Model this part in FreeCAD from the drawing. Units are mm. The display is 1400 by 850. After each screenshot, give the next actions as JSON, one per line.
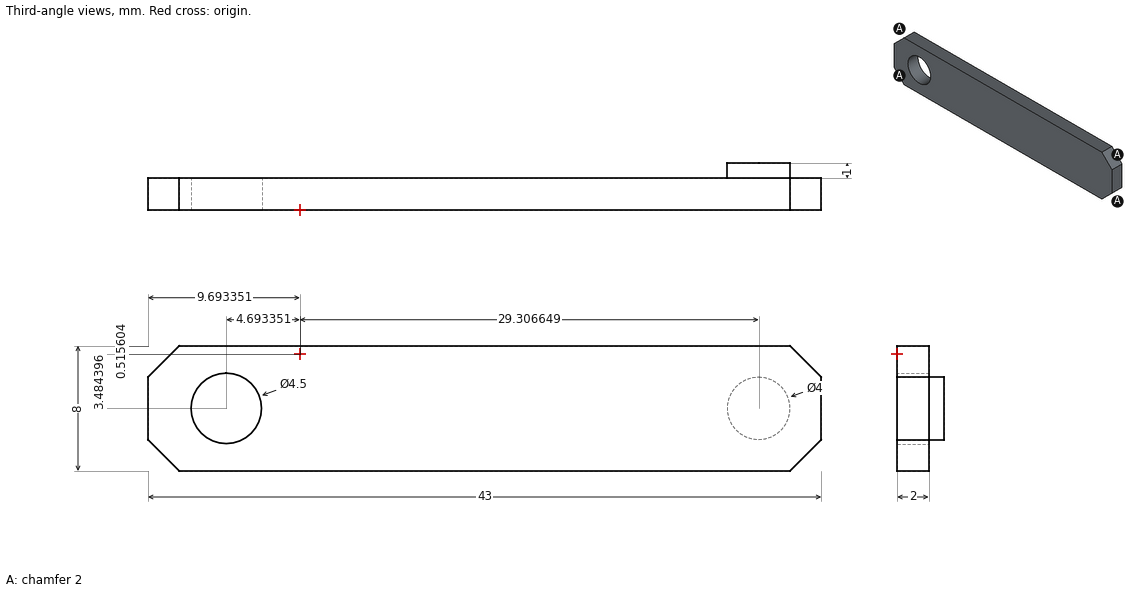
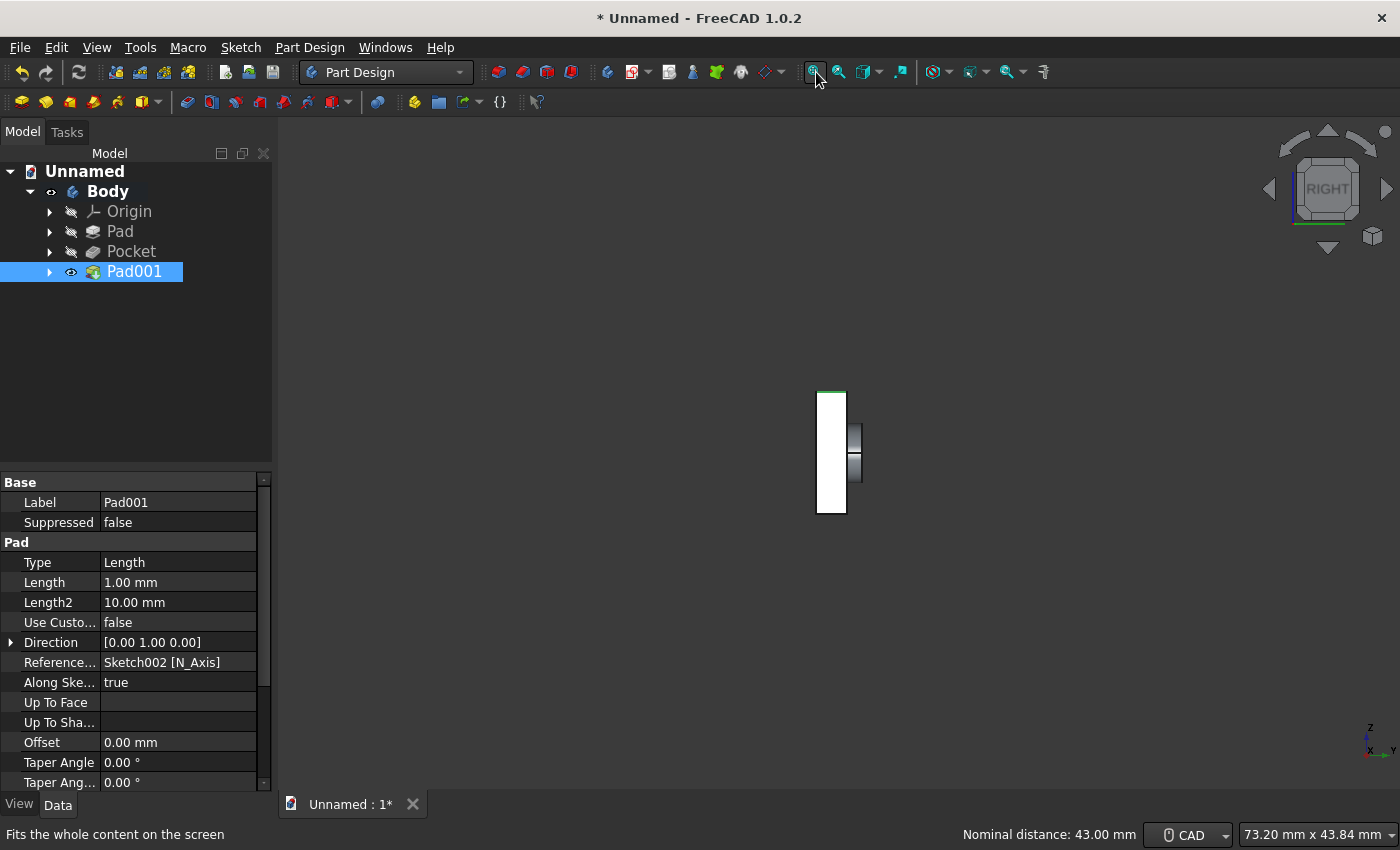
{"action": "left_click", "coordinate": [831, 513], "text": "ctrl"}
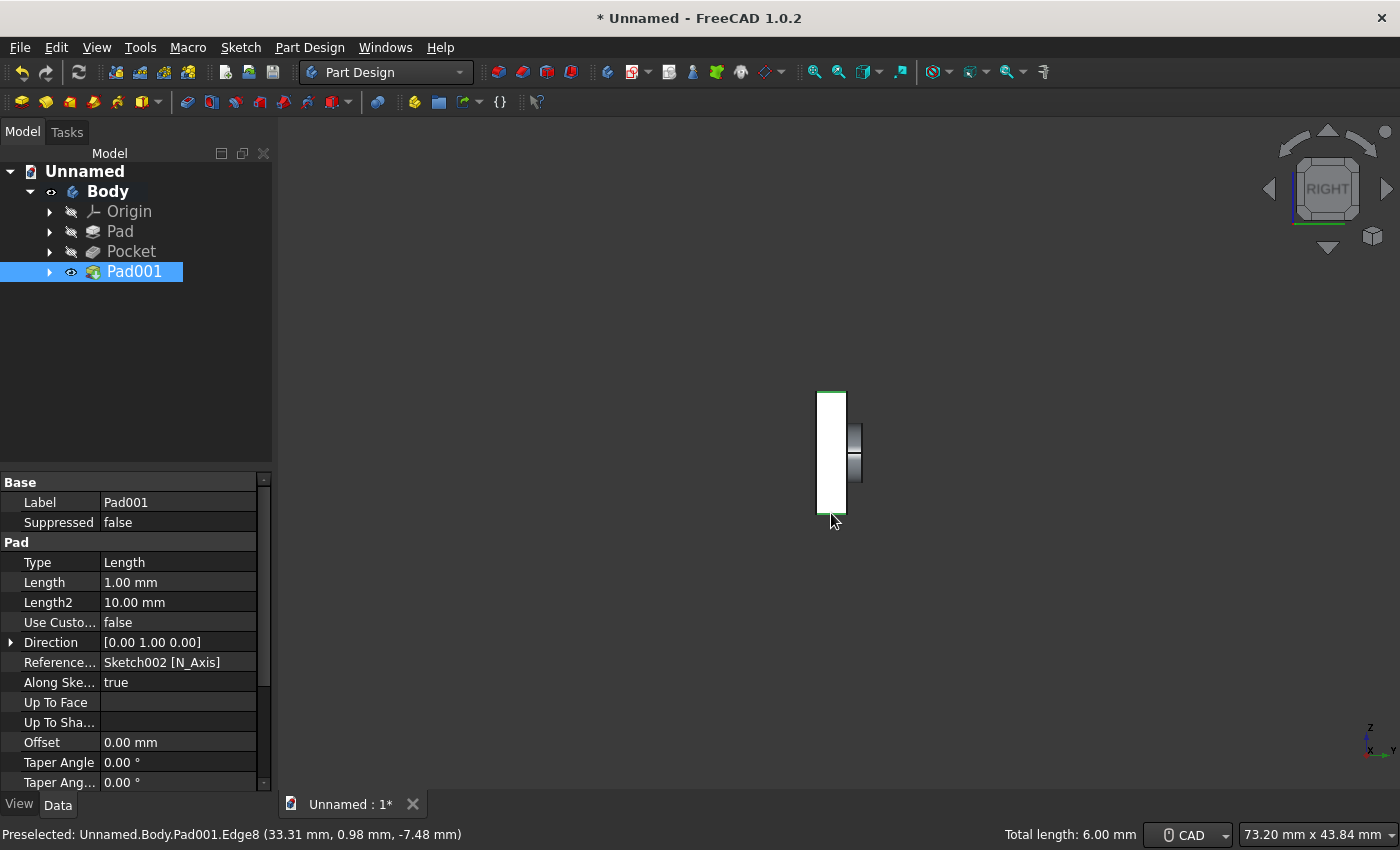
{"action": "key", "text": "5"}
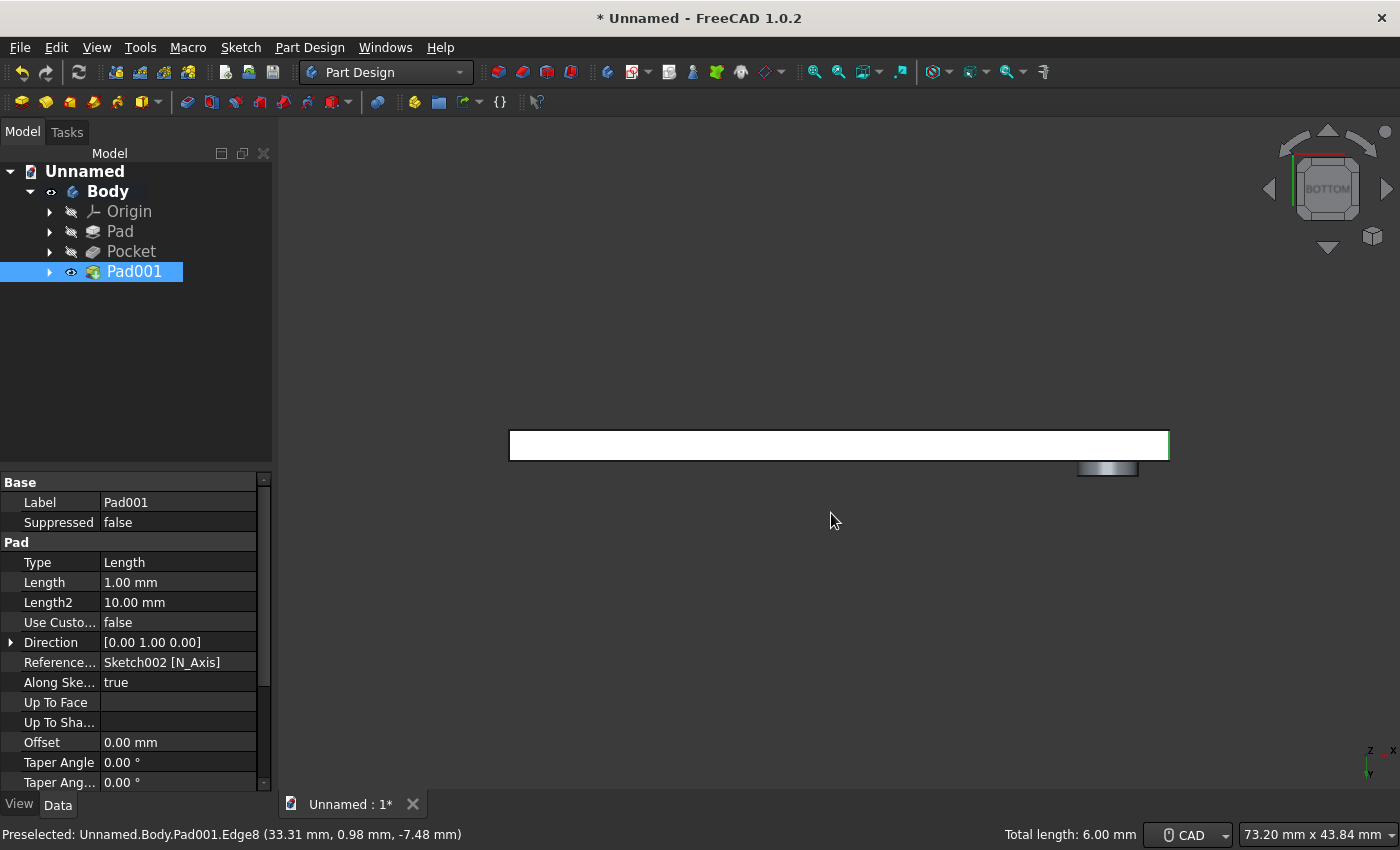
{"action": "left_click", "coordinate": [509, 444], "text": "ctrl"}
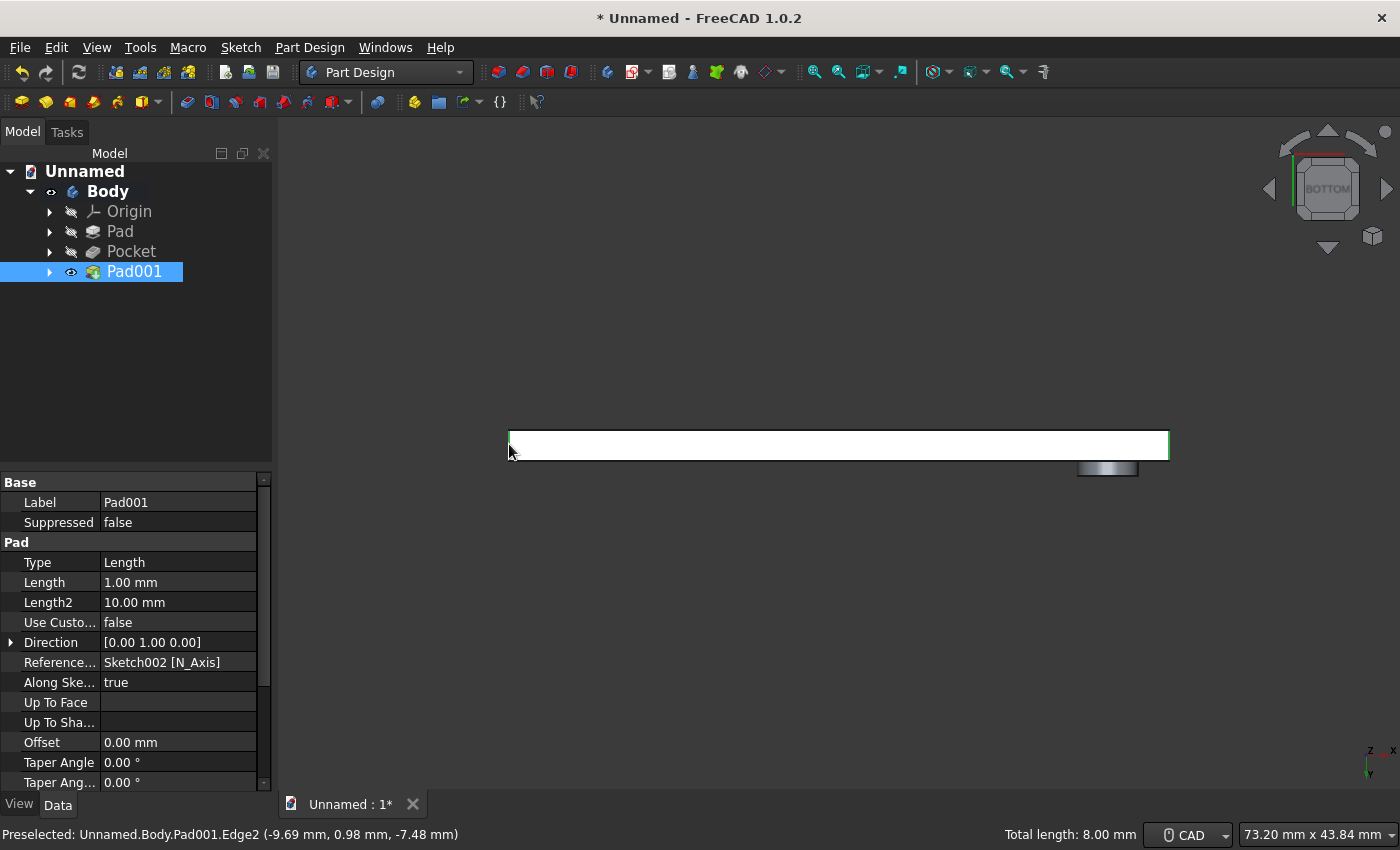
{"action": "left_click", "coordinate": [524, 72]}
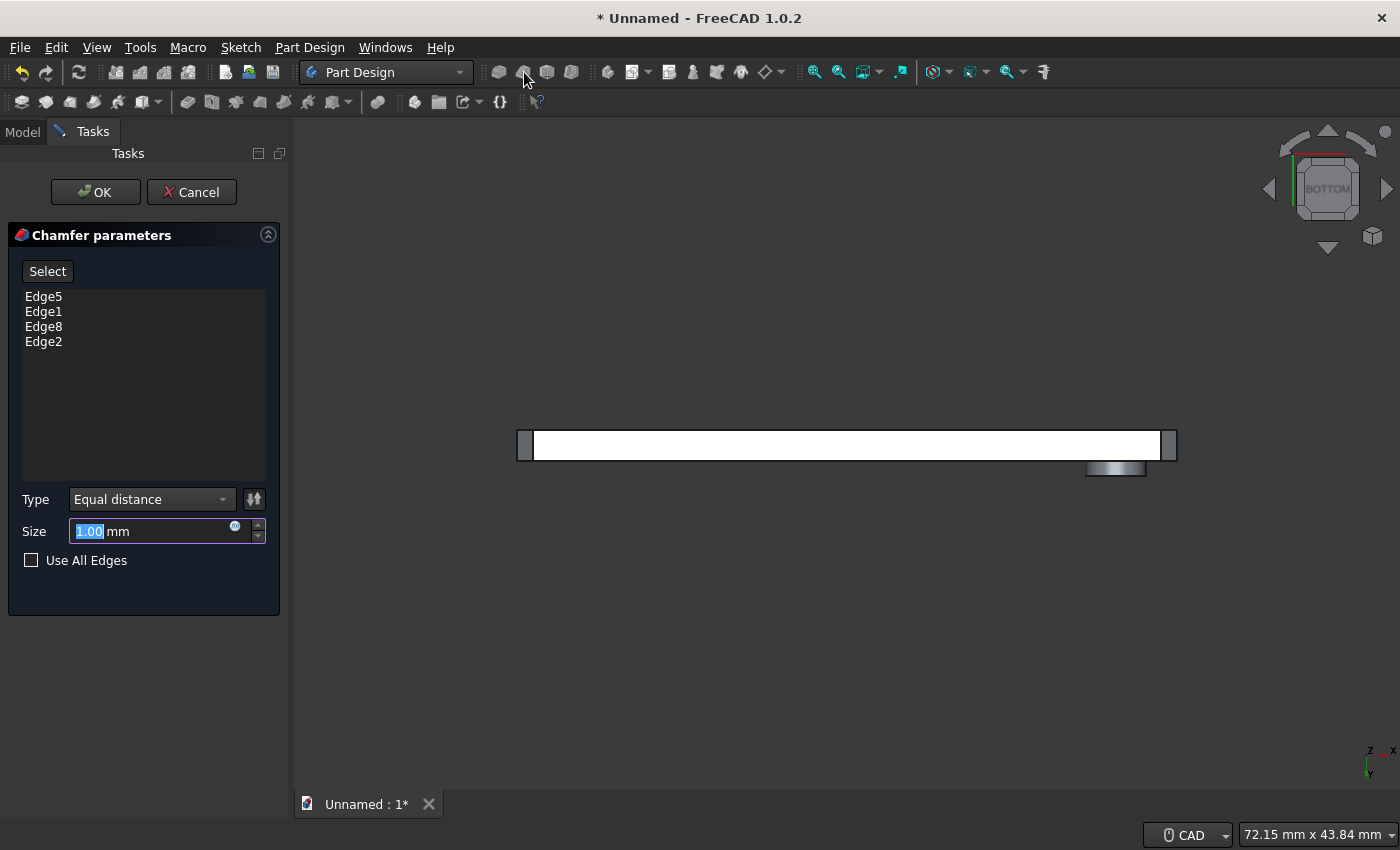
{"action": "type", "text": "2"}
{"action": "key", "text": "Tab"}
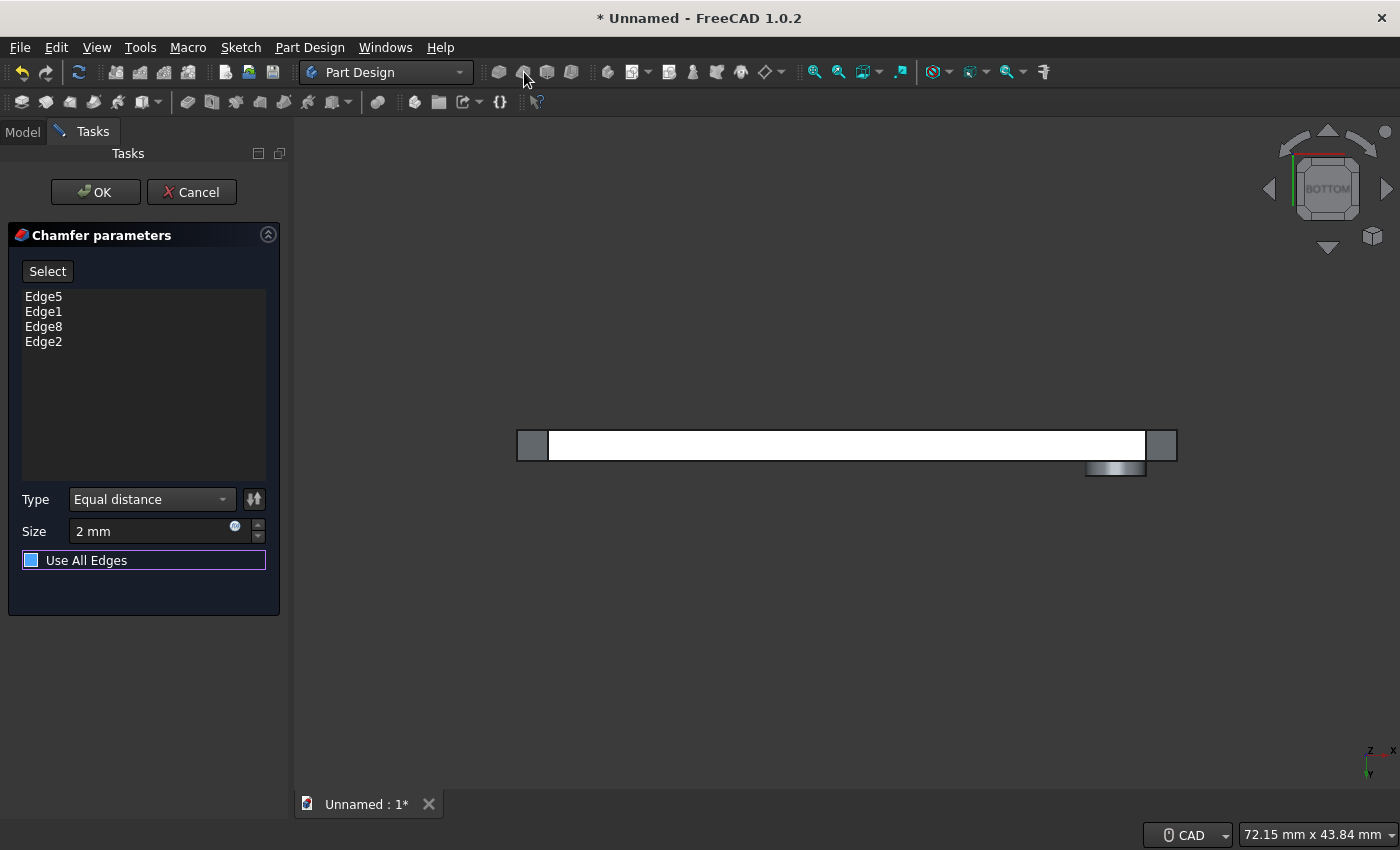
{"action": "left_click", "coordinate": [96, 192]}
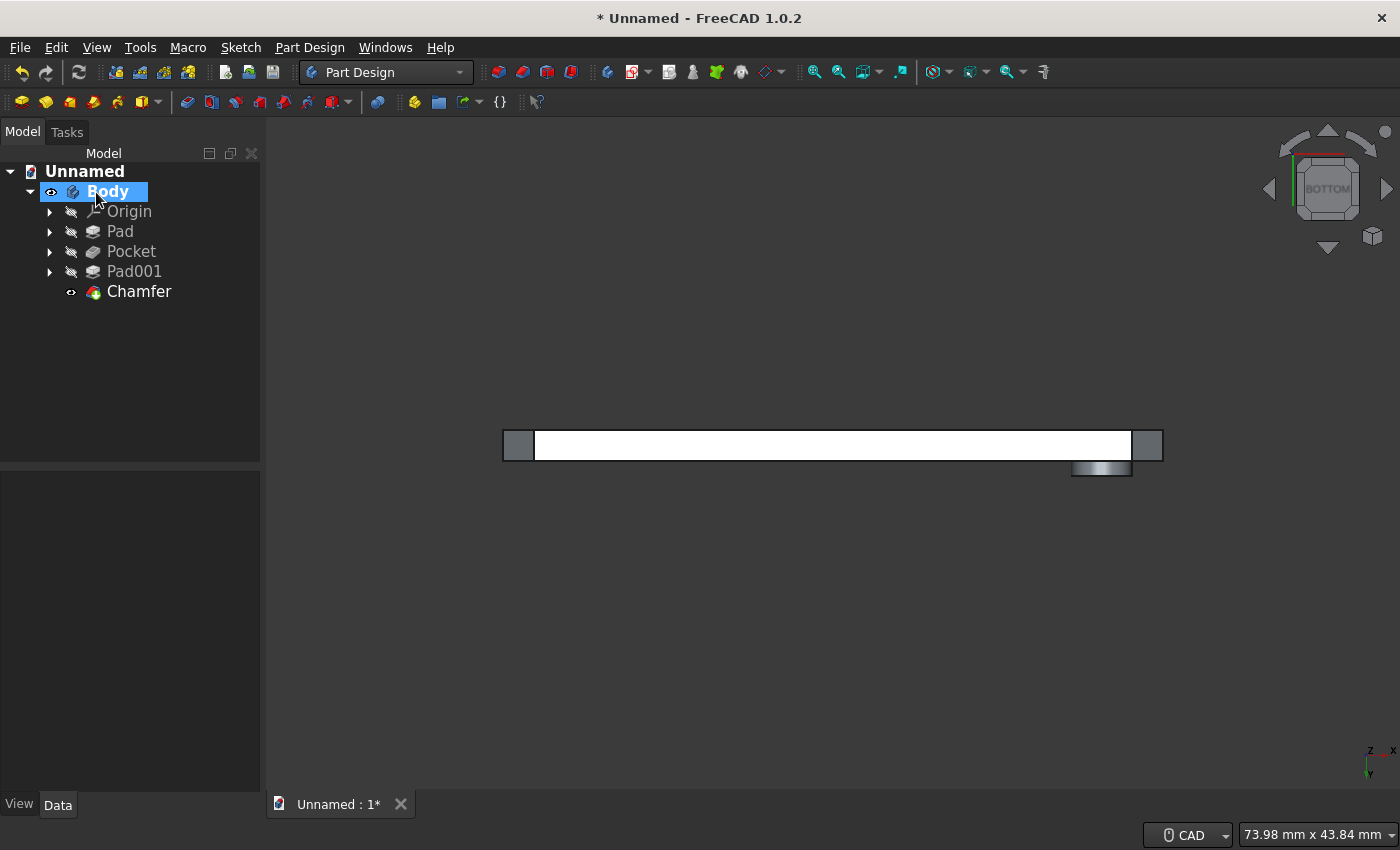
{"action": "key", "text": "0"}